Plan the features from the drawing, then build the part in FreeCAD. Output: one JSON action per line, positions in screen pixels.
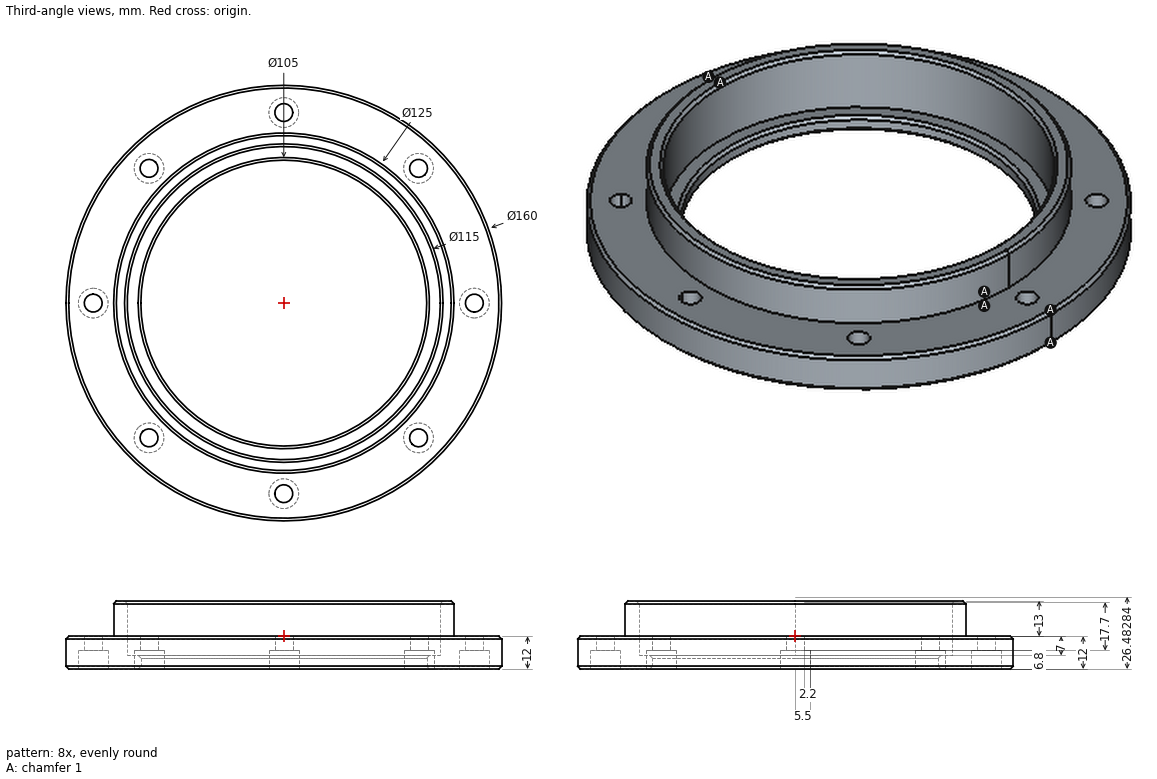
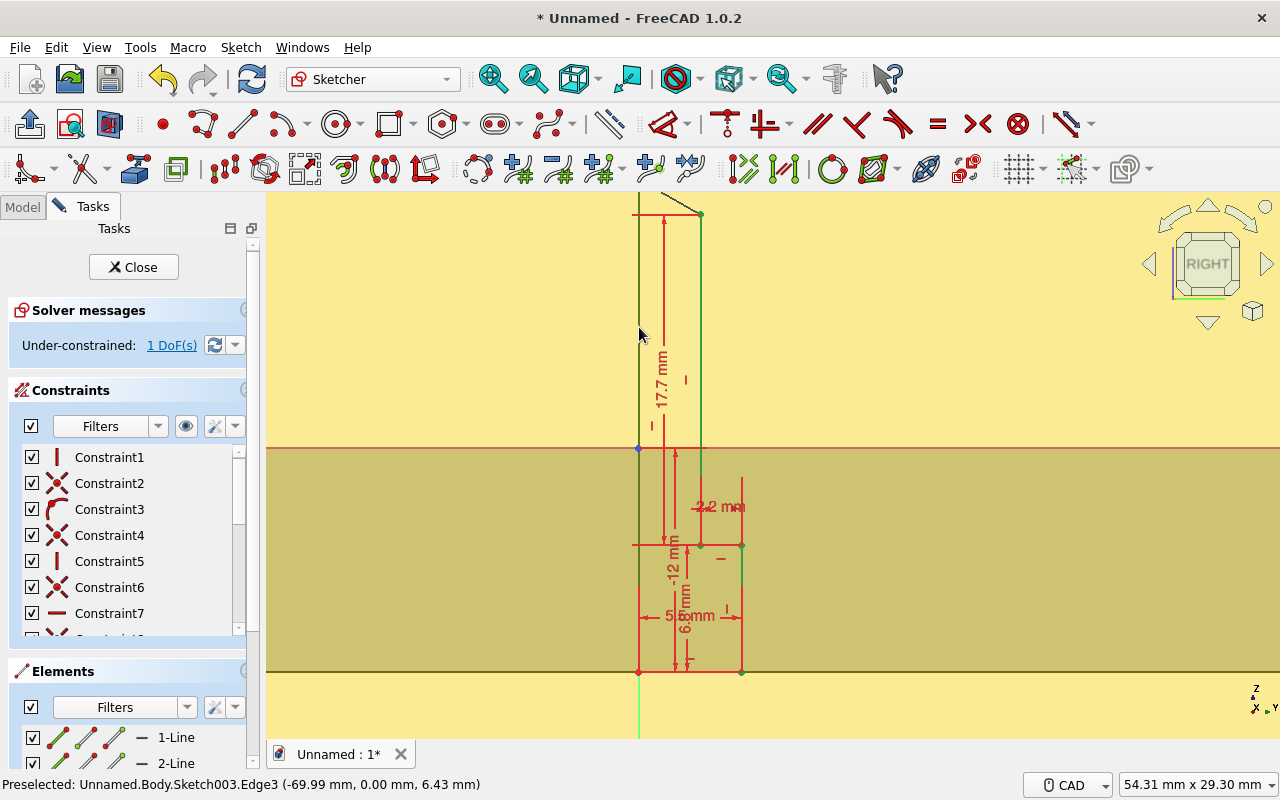
{"action": "key", "text": "i"}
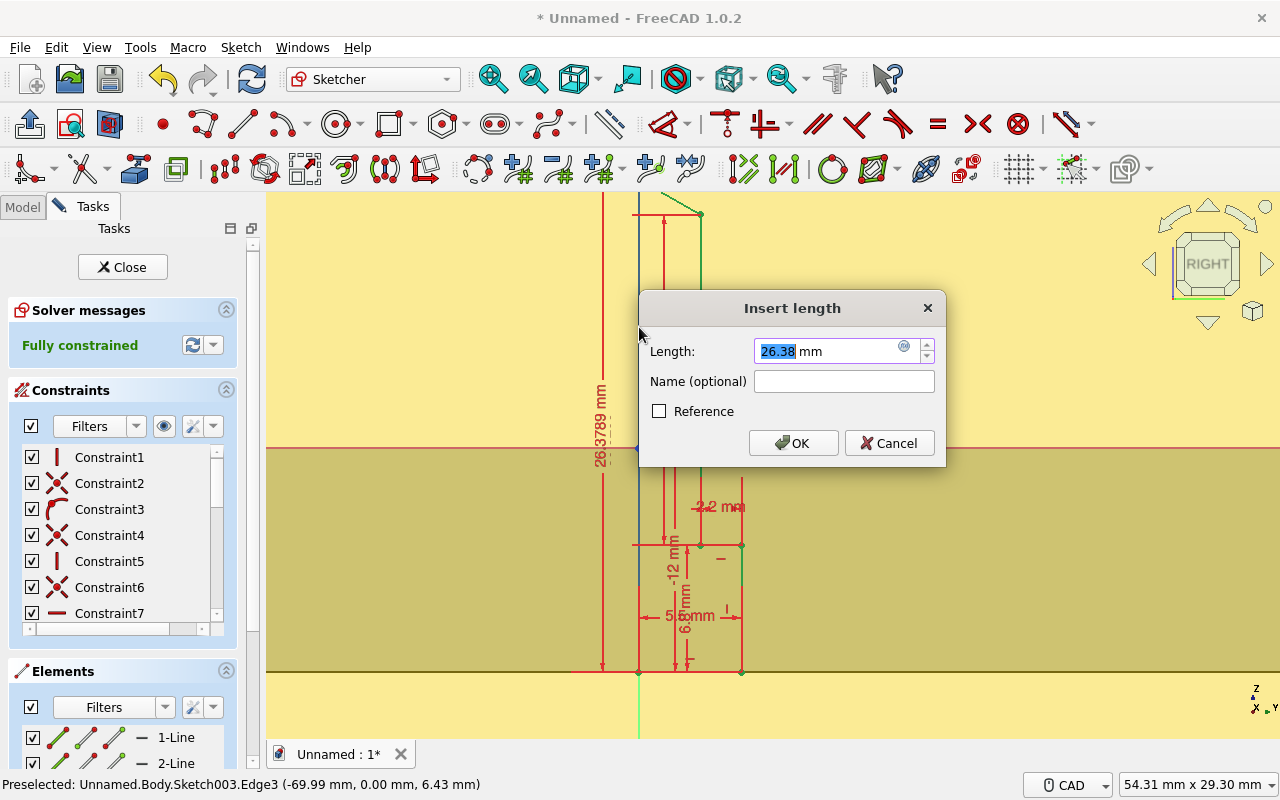
{"action": "type", "text": "26.48284"}
{"action": "key", "text": "Return"}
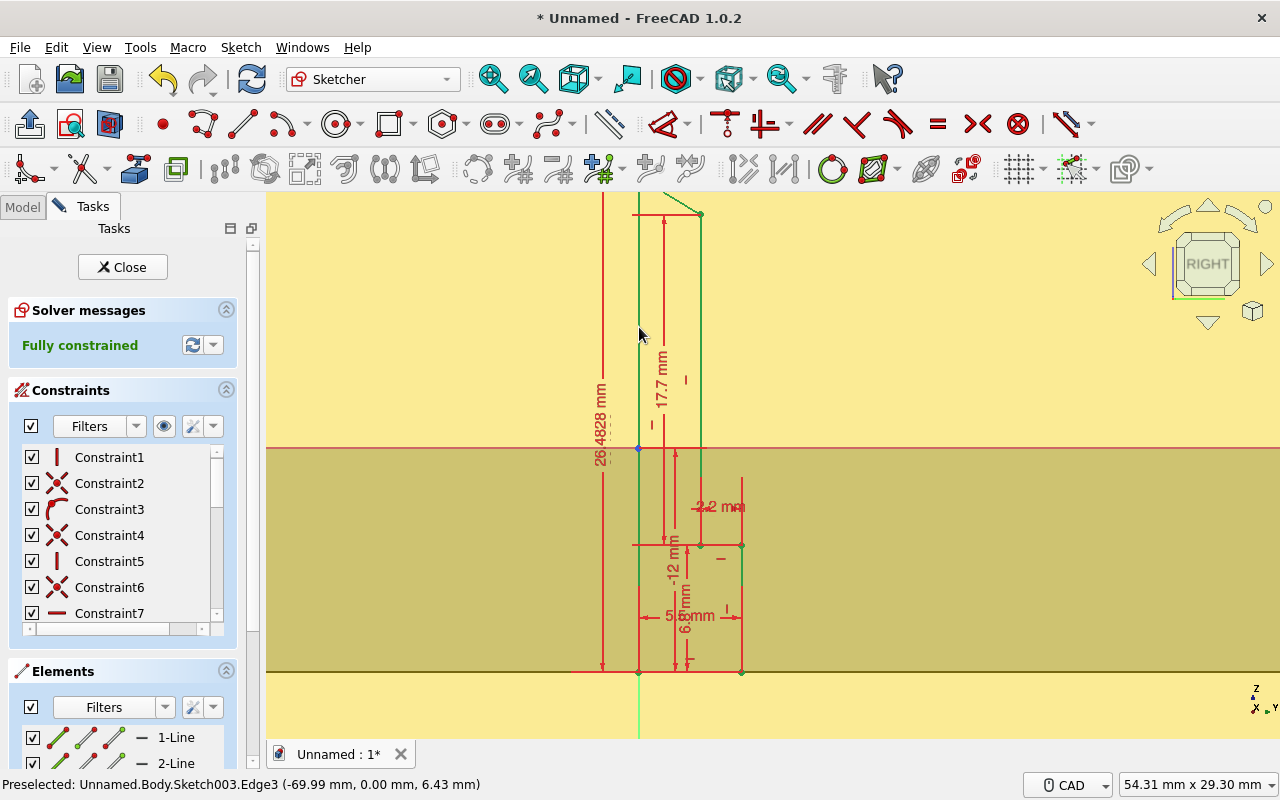
{"action": "left_click", "coordinate": [123, 267]}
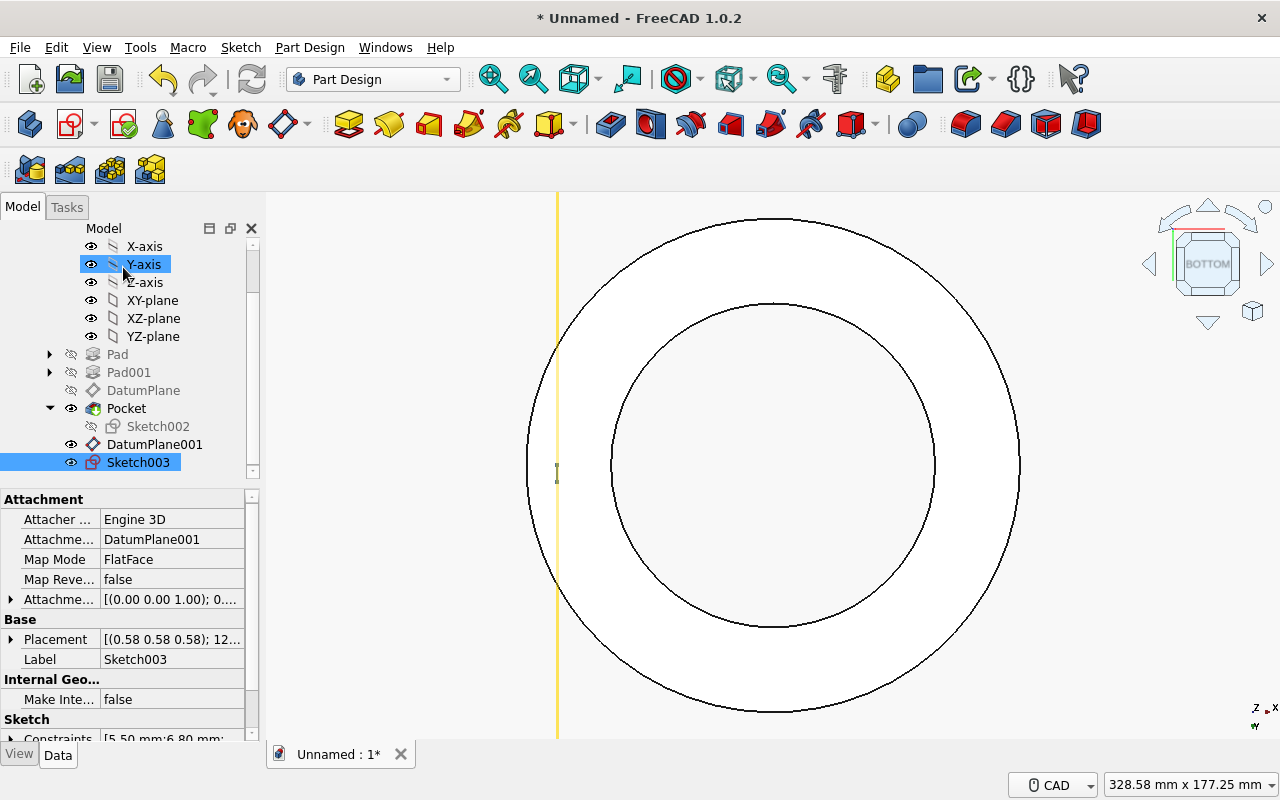
{"action": "left_click", "coordinate": [692, 124]}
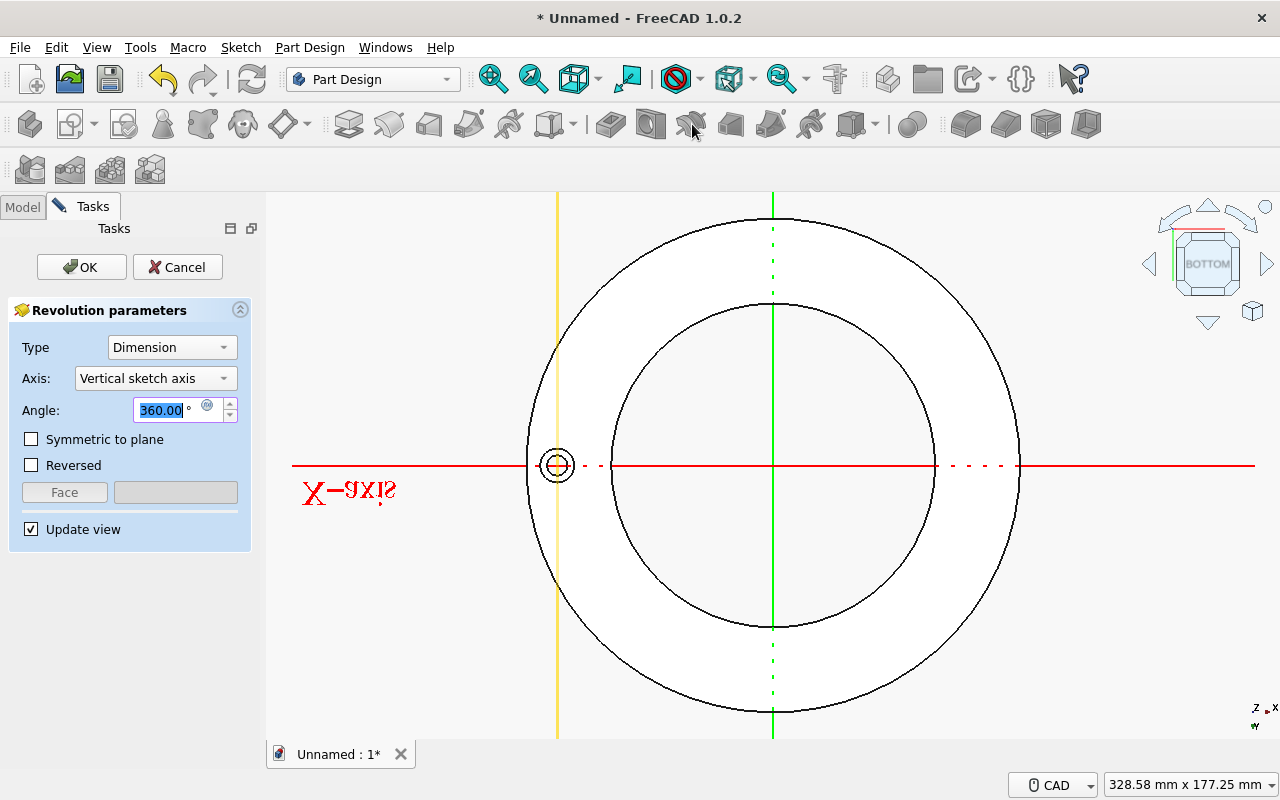
{"action": "left_click", "coordinate": [82, 267]}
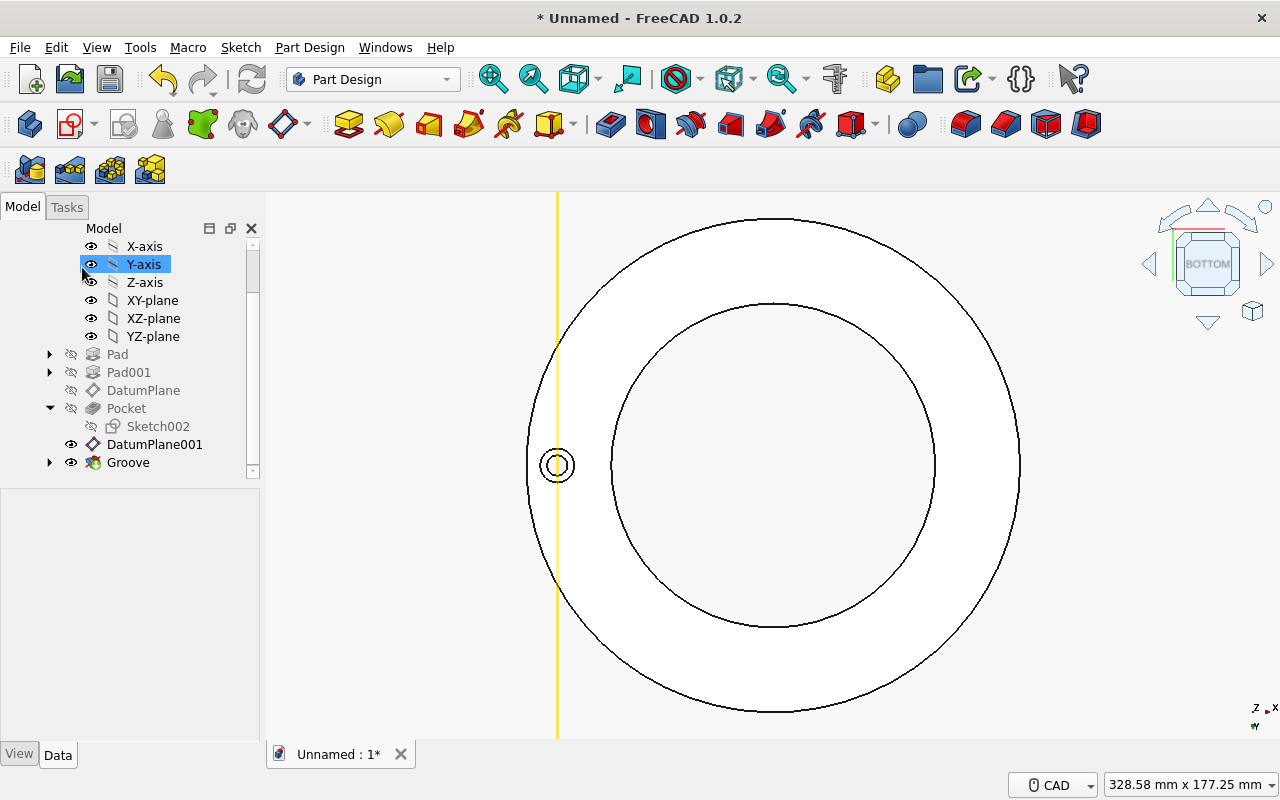
{"action": "left_click", "coordinate": [116, 444]}
{"action": "key", "text": "space"}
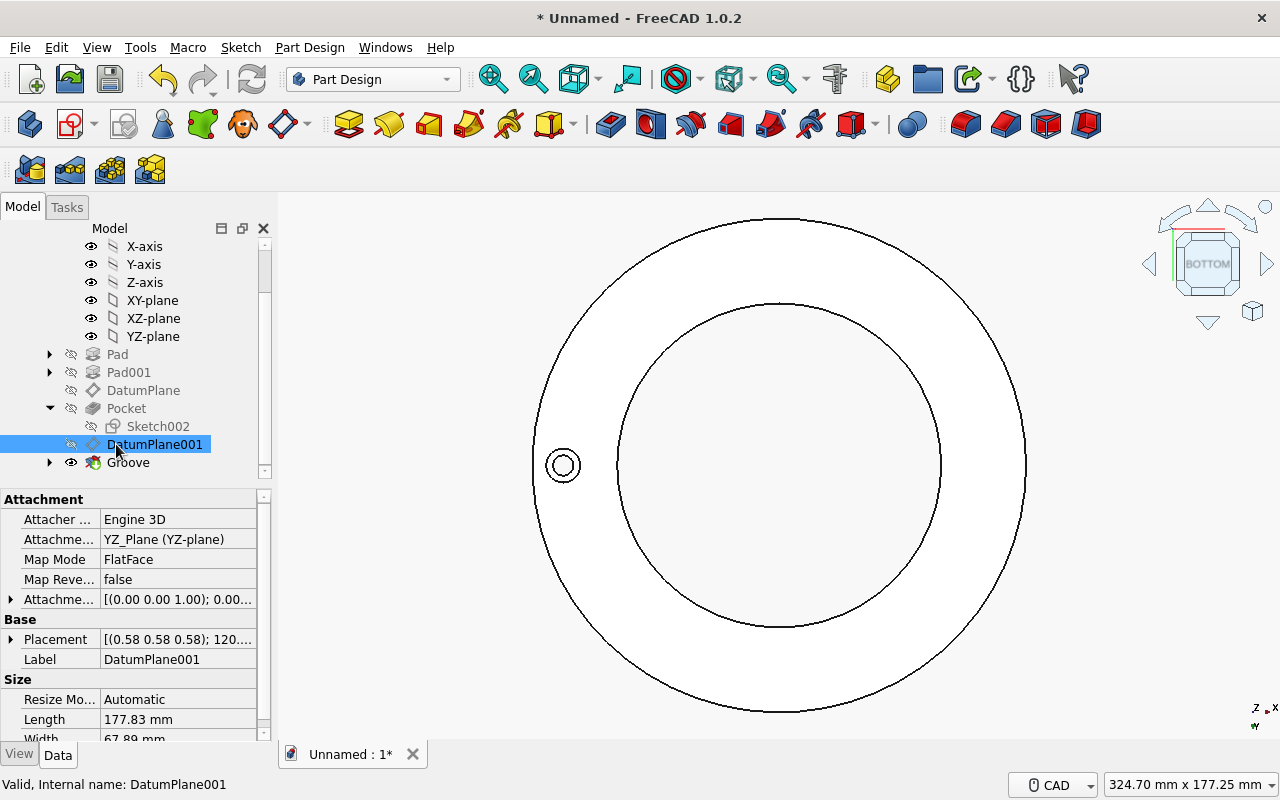
{"action": "left_click", "coordinate": [116, 462]}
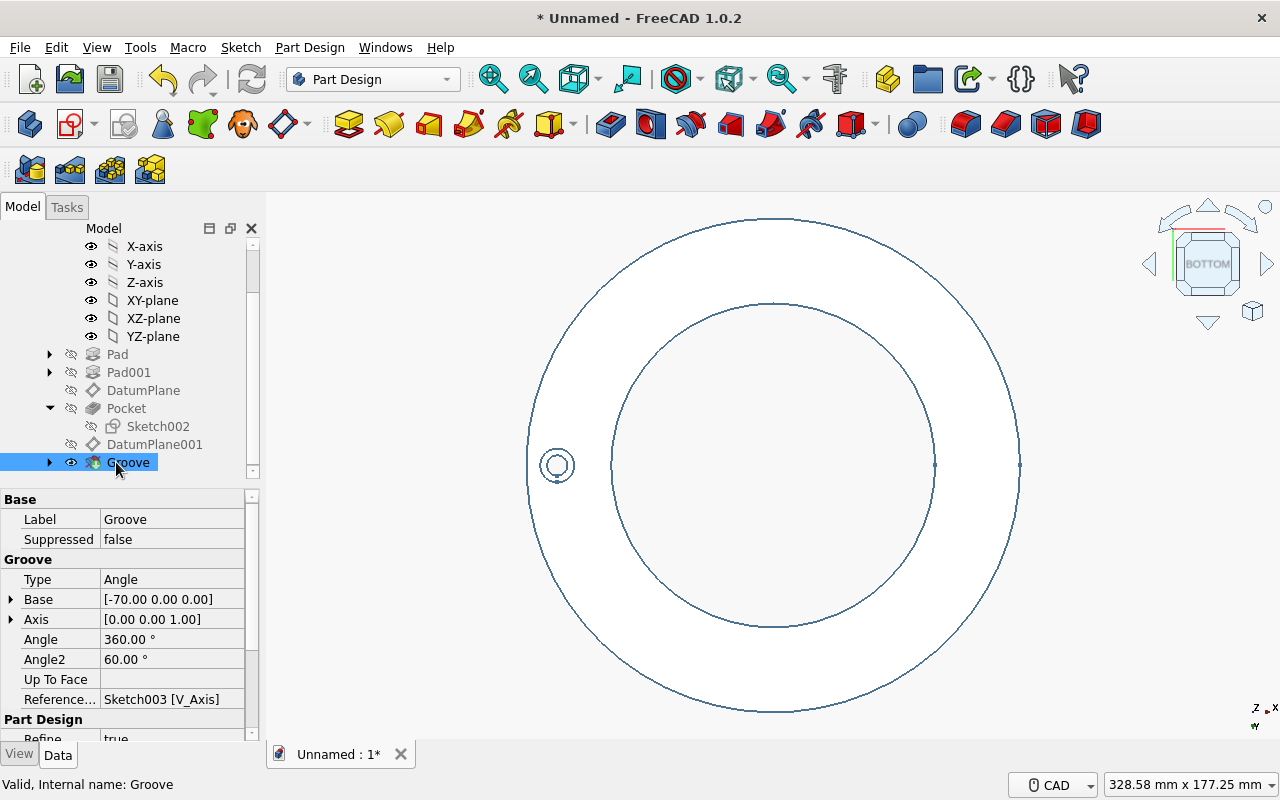
{"action": "left_click", "coordinate": [110, 170]}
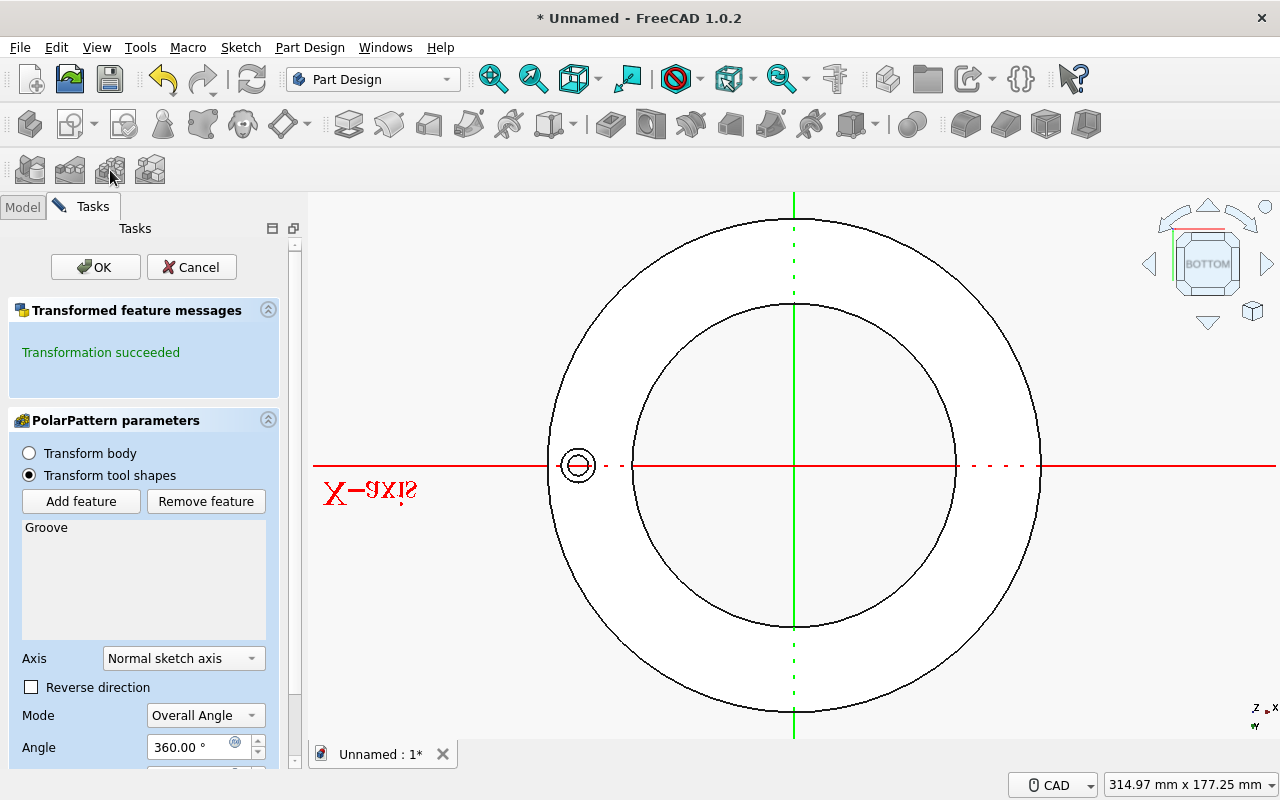
{"action": "left_click", "coordinate": [184, 658]}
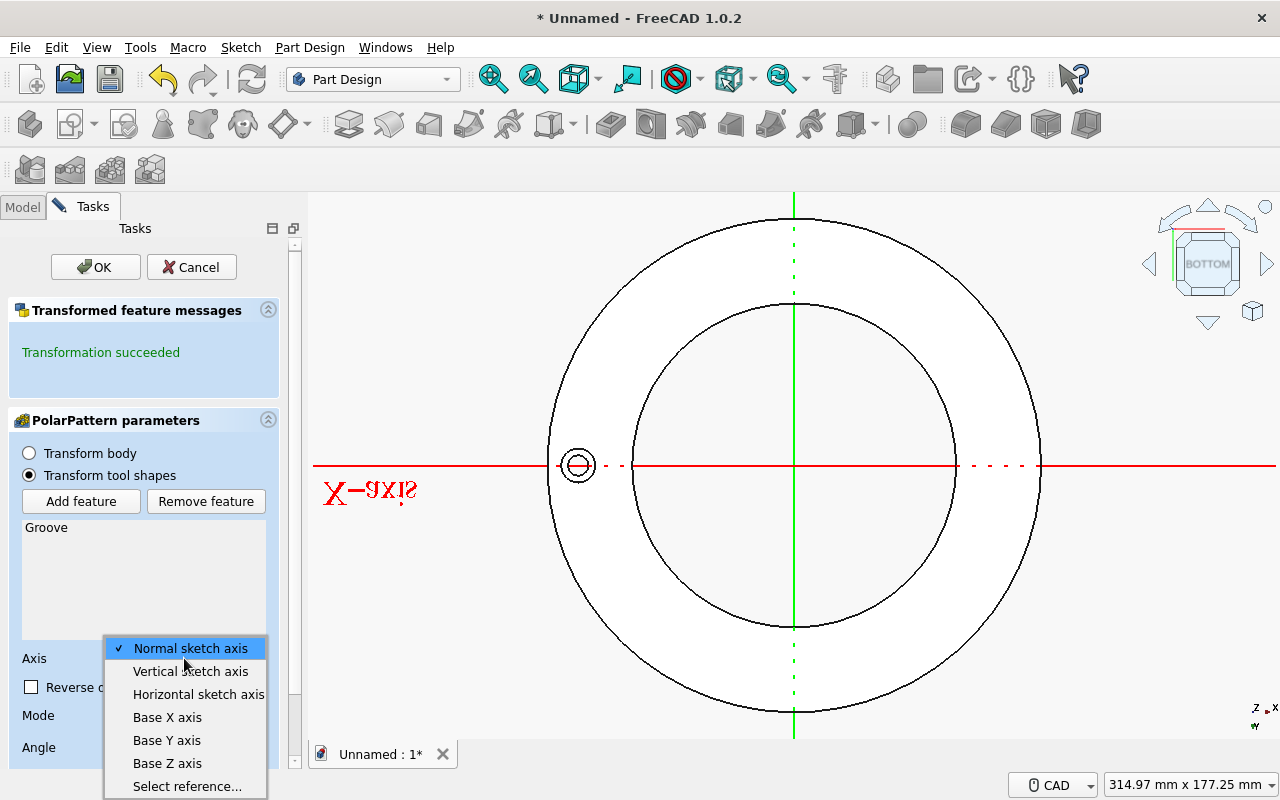
{"action": "left_click", "coordinate": [184, 764]}